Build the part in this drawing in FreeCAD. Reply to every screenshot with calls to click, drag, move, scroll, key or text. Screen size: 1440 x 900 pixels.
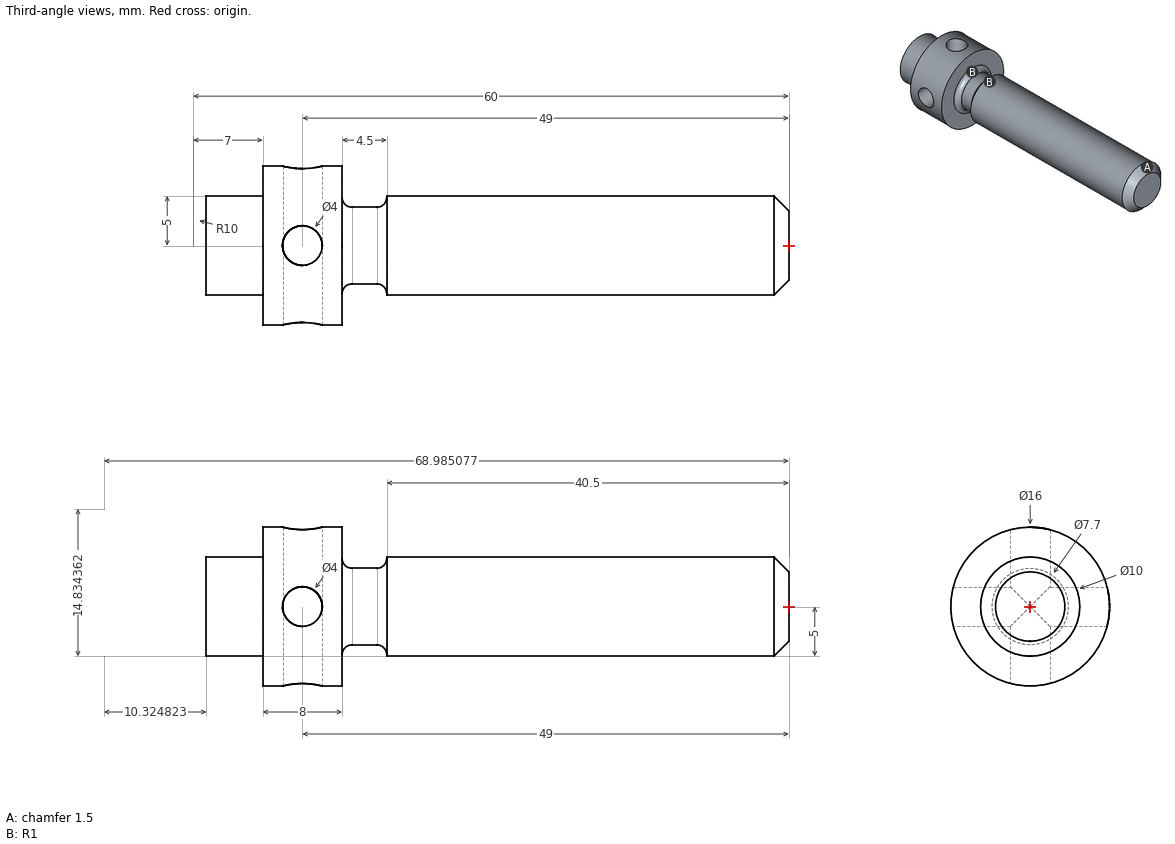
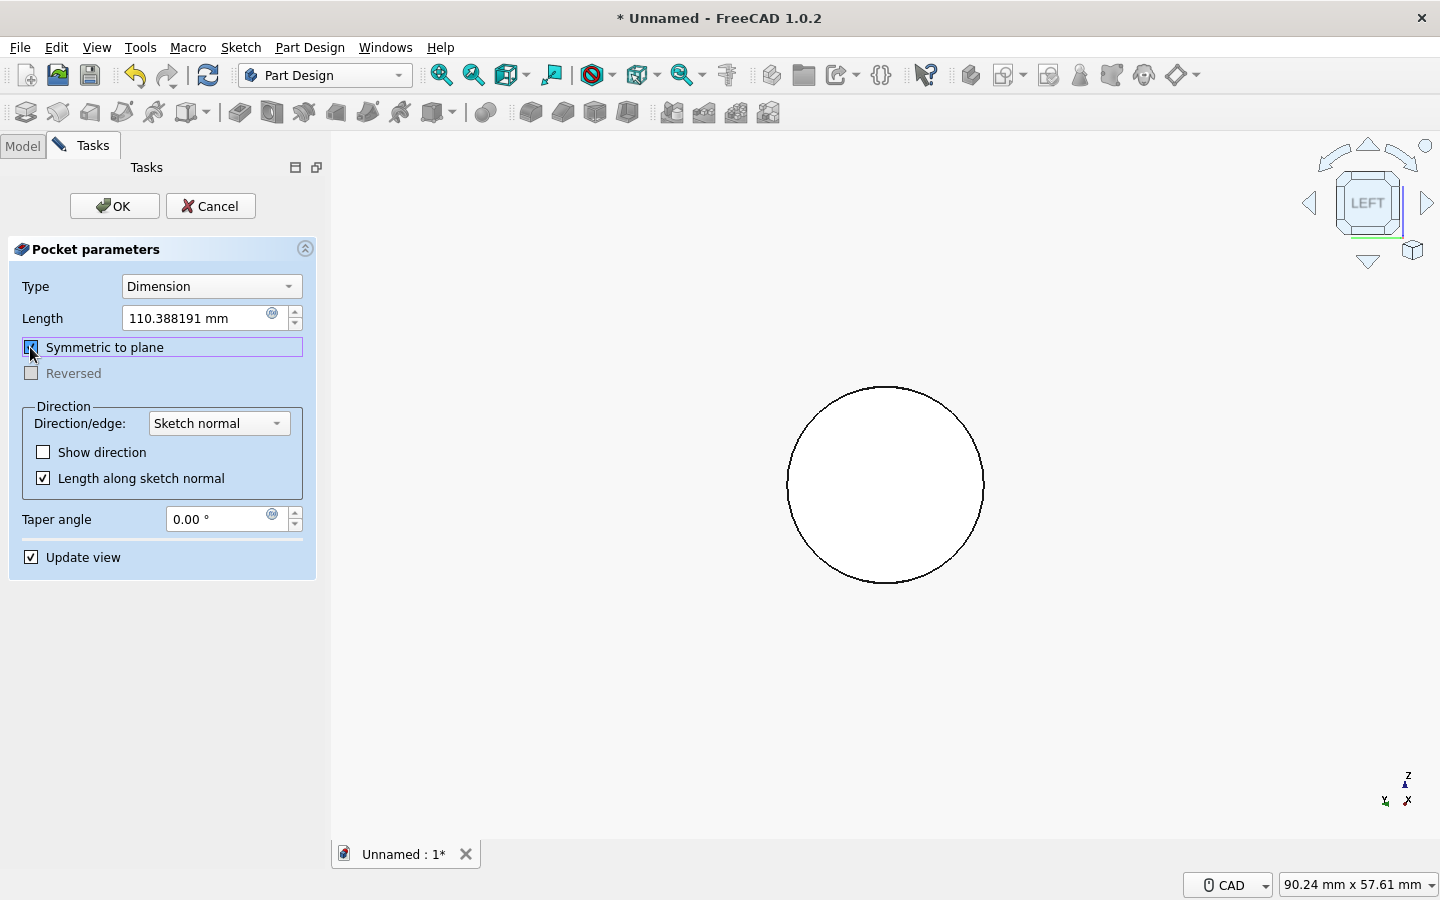
click(115, 206)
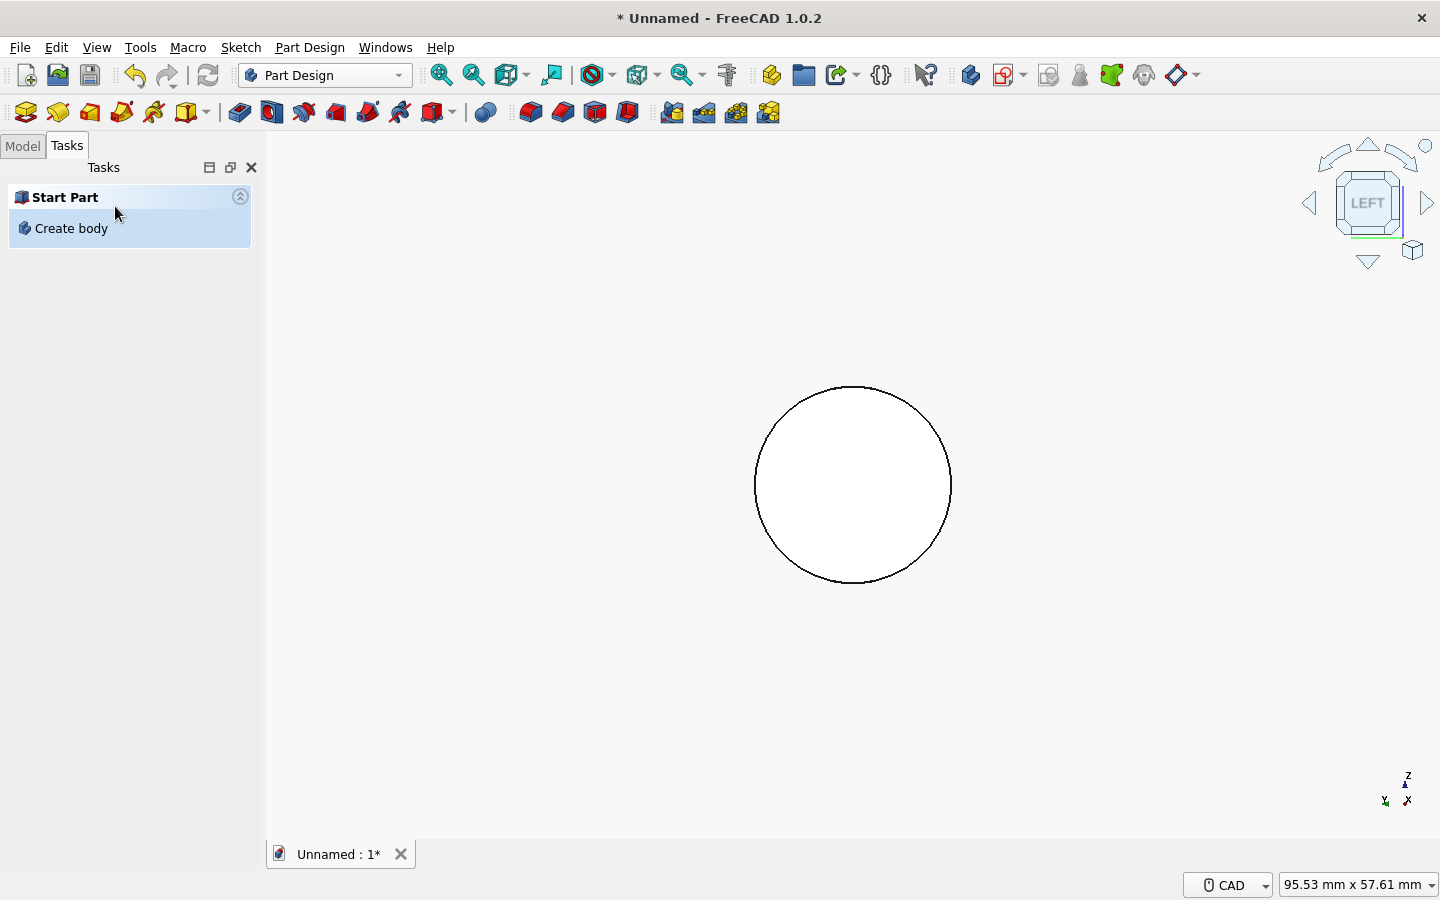
key(v)
key(f)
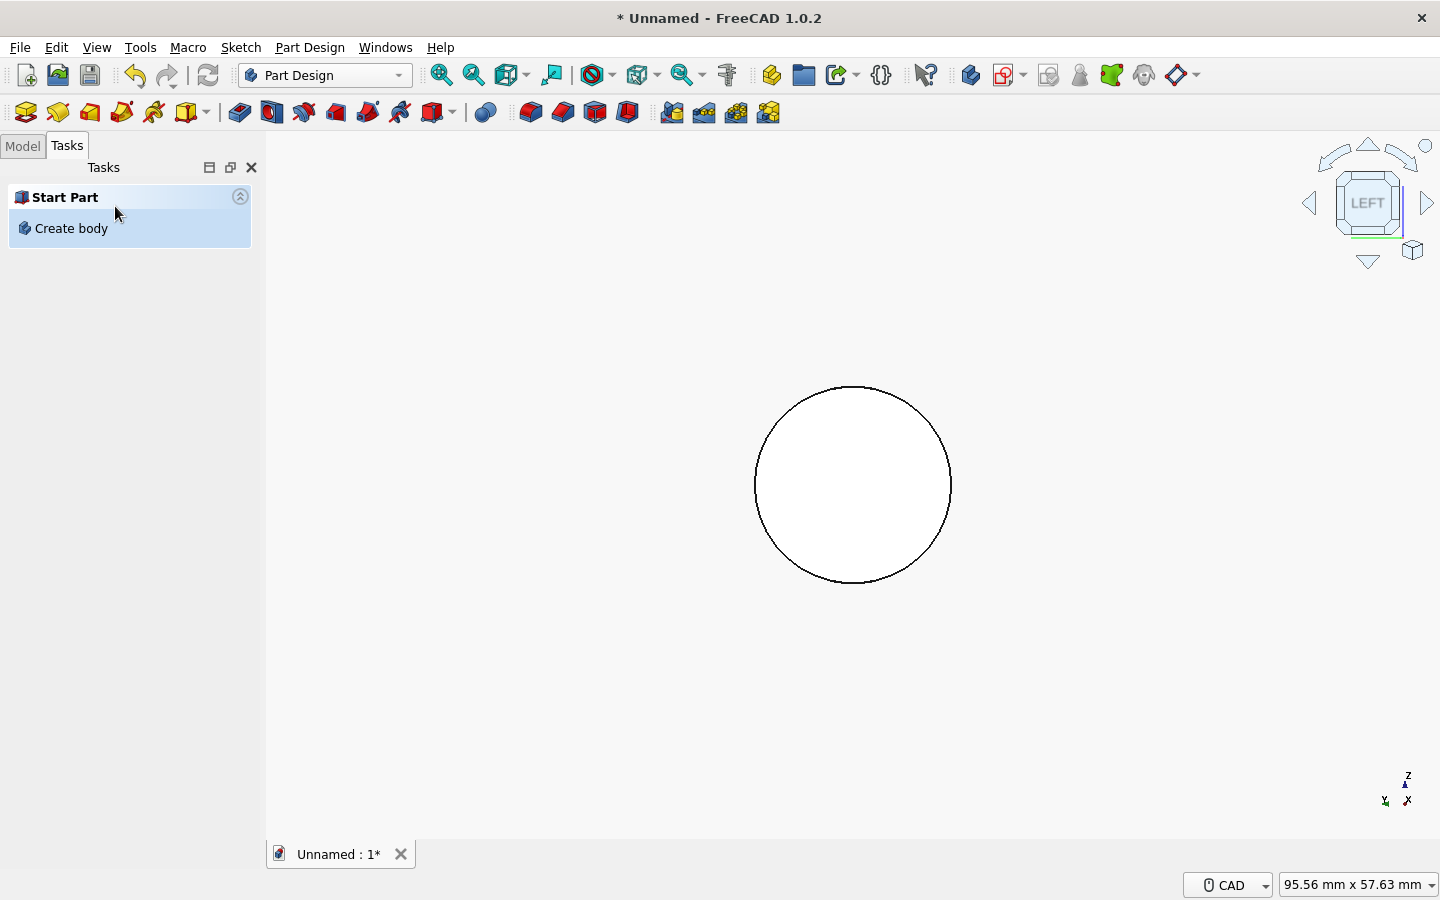
click(1004, 76)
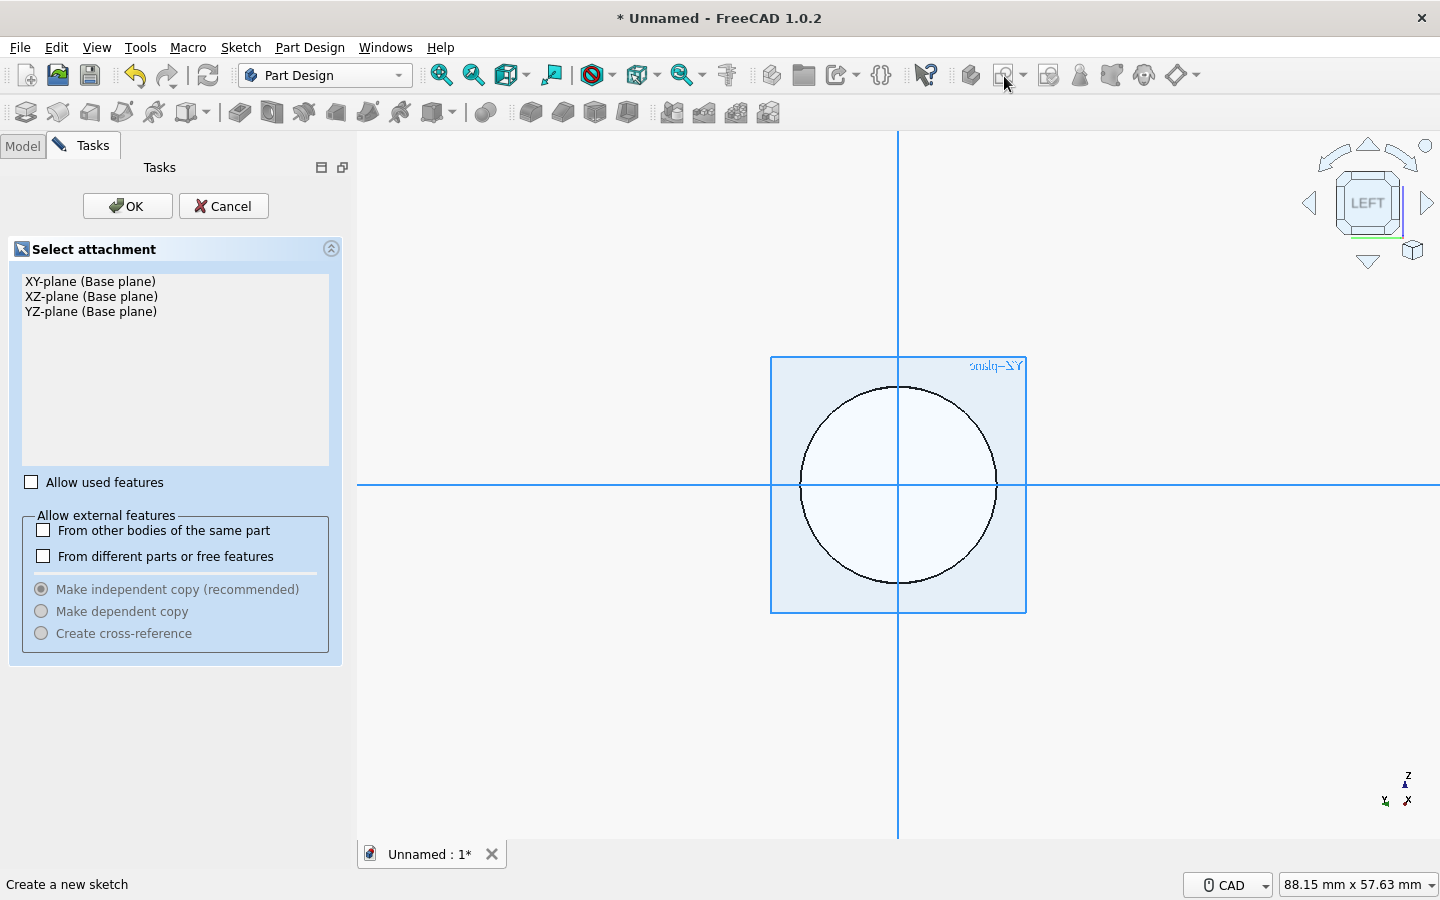
click(82, 296)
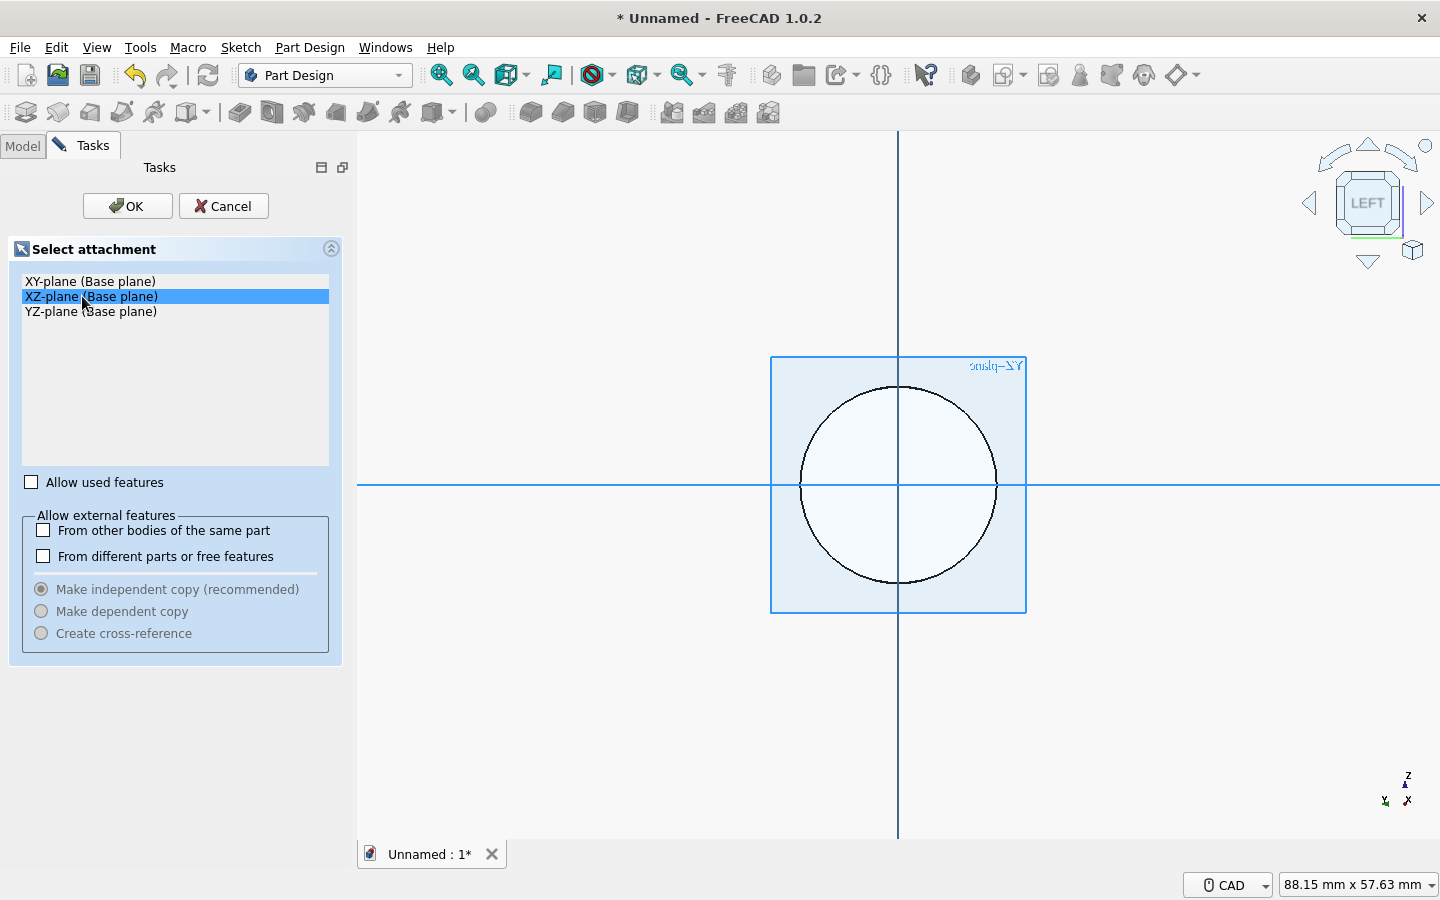
click(128, 206)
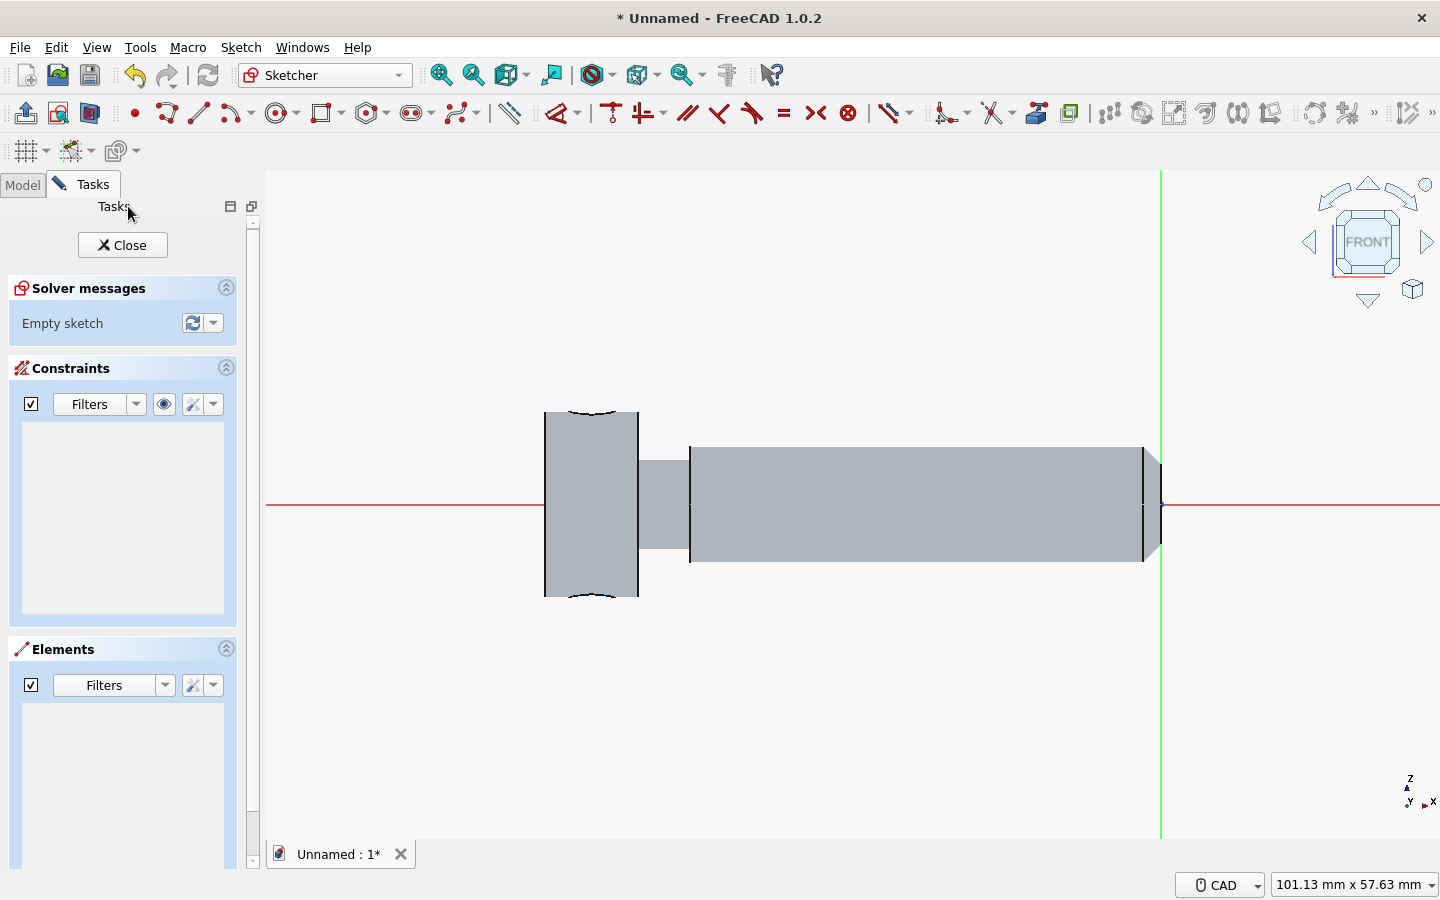
key(q)
key(s)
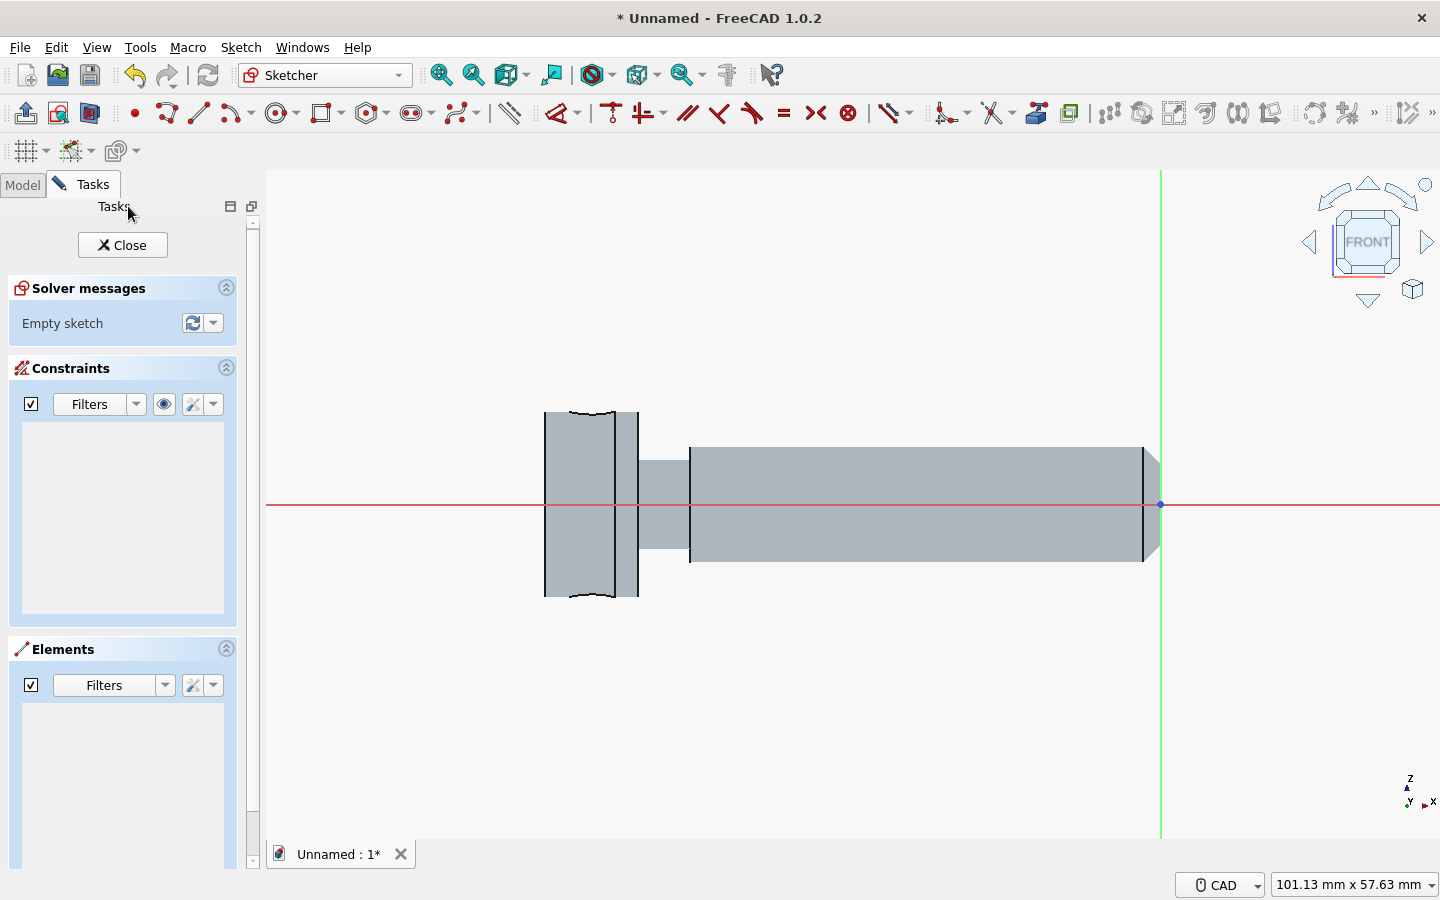
scroll(568, 504, up, 11)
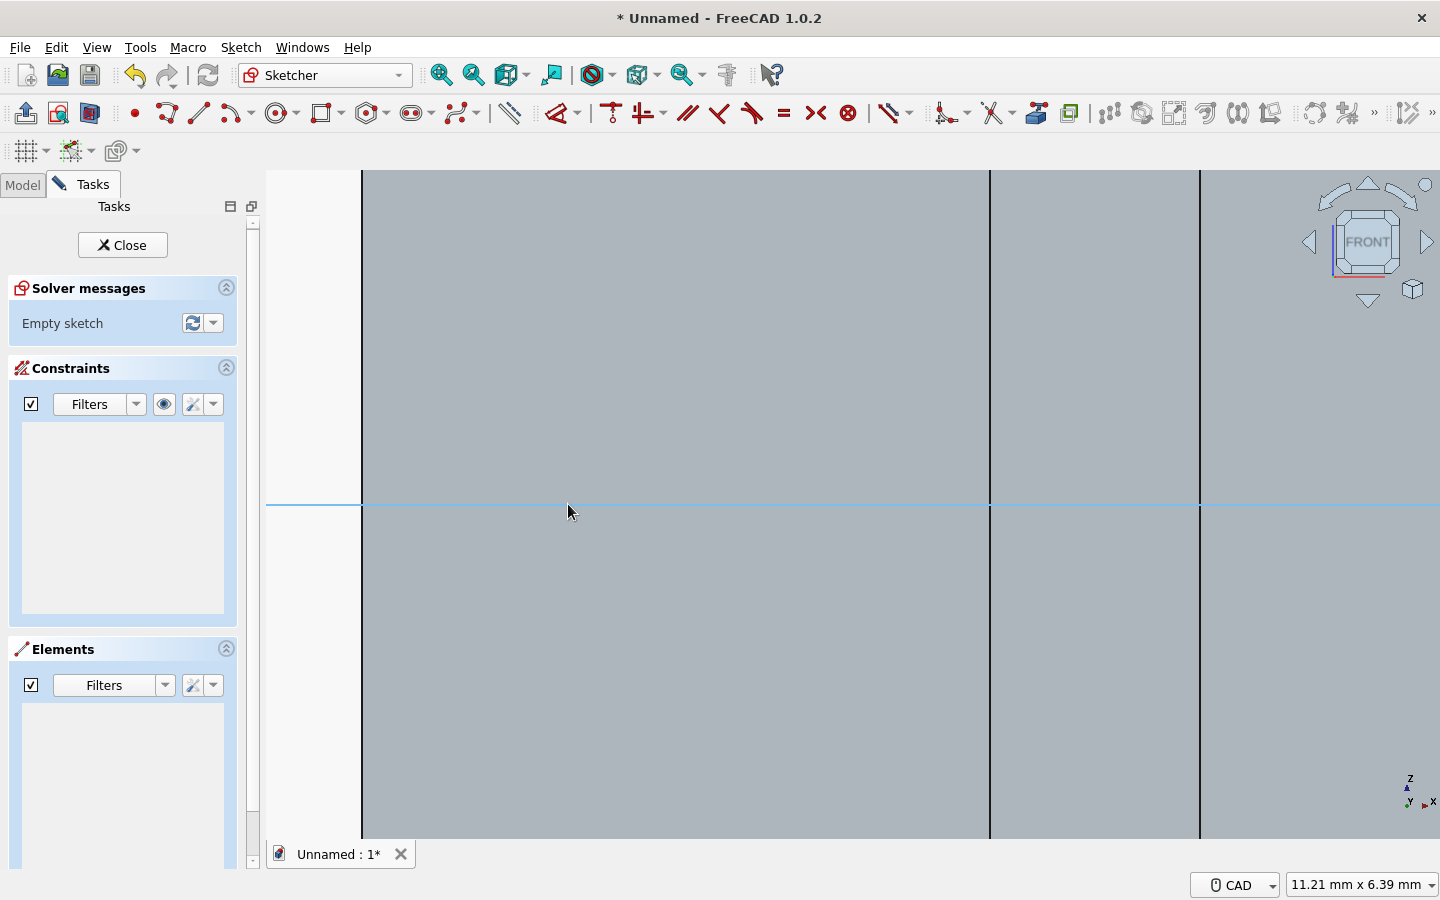
click(276, 114)